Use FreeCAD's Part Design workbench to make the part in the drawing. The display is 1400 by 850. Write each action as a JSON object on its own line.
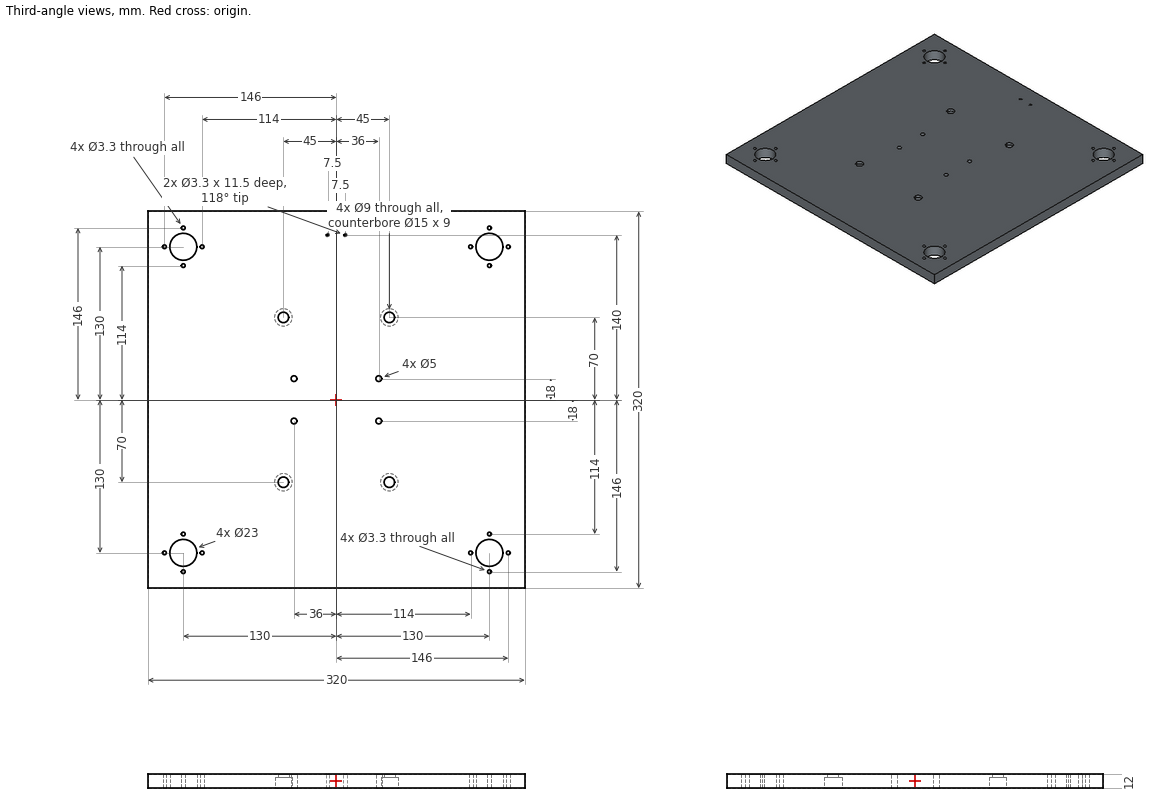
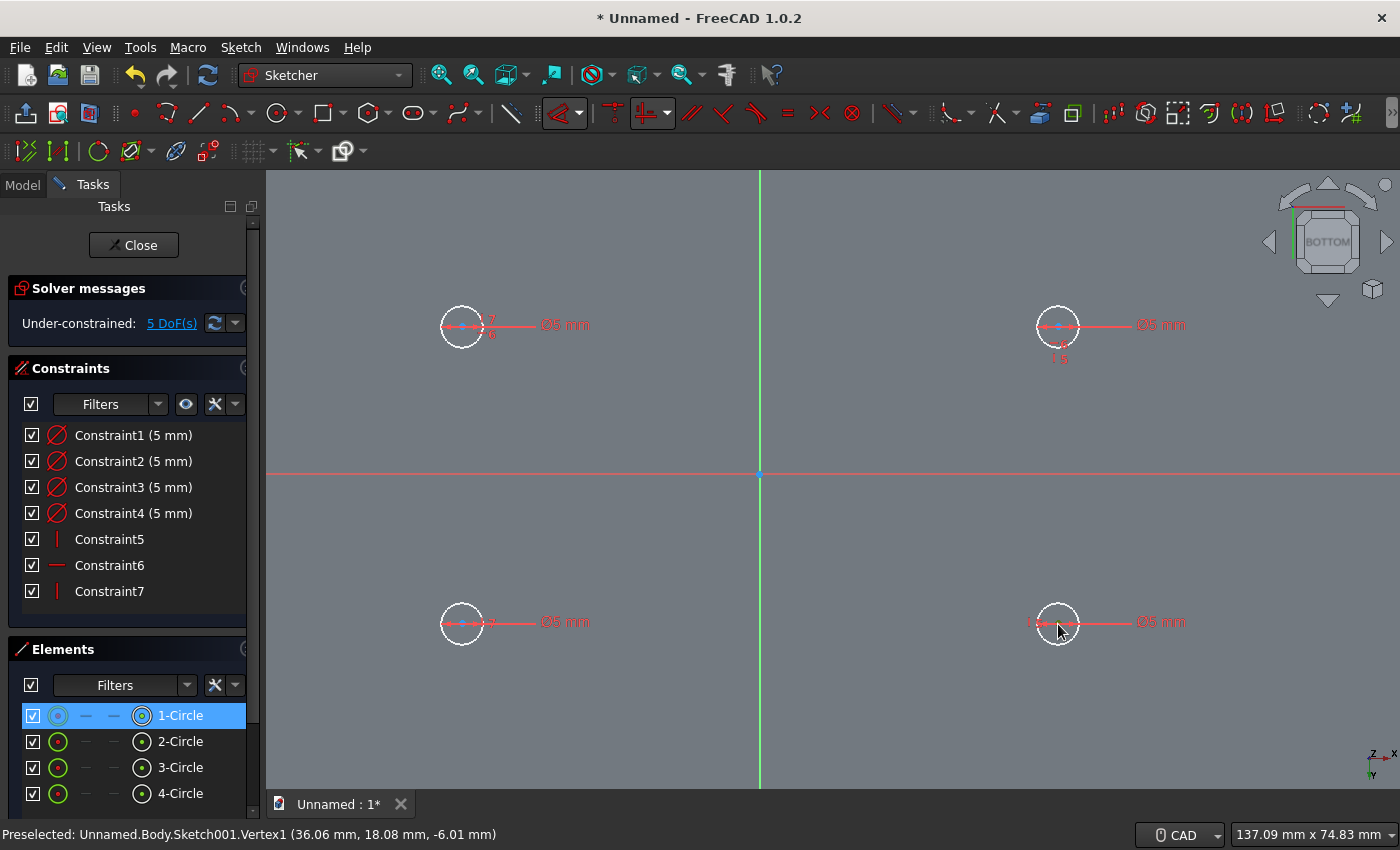
{"action": "left_click", "coordinate": [462, 624]}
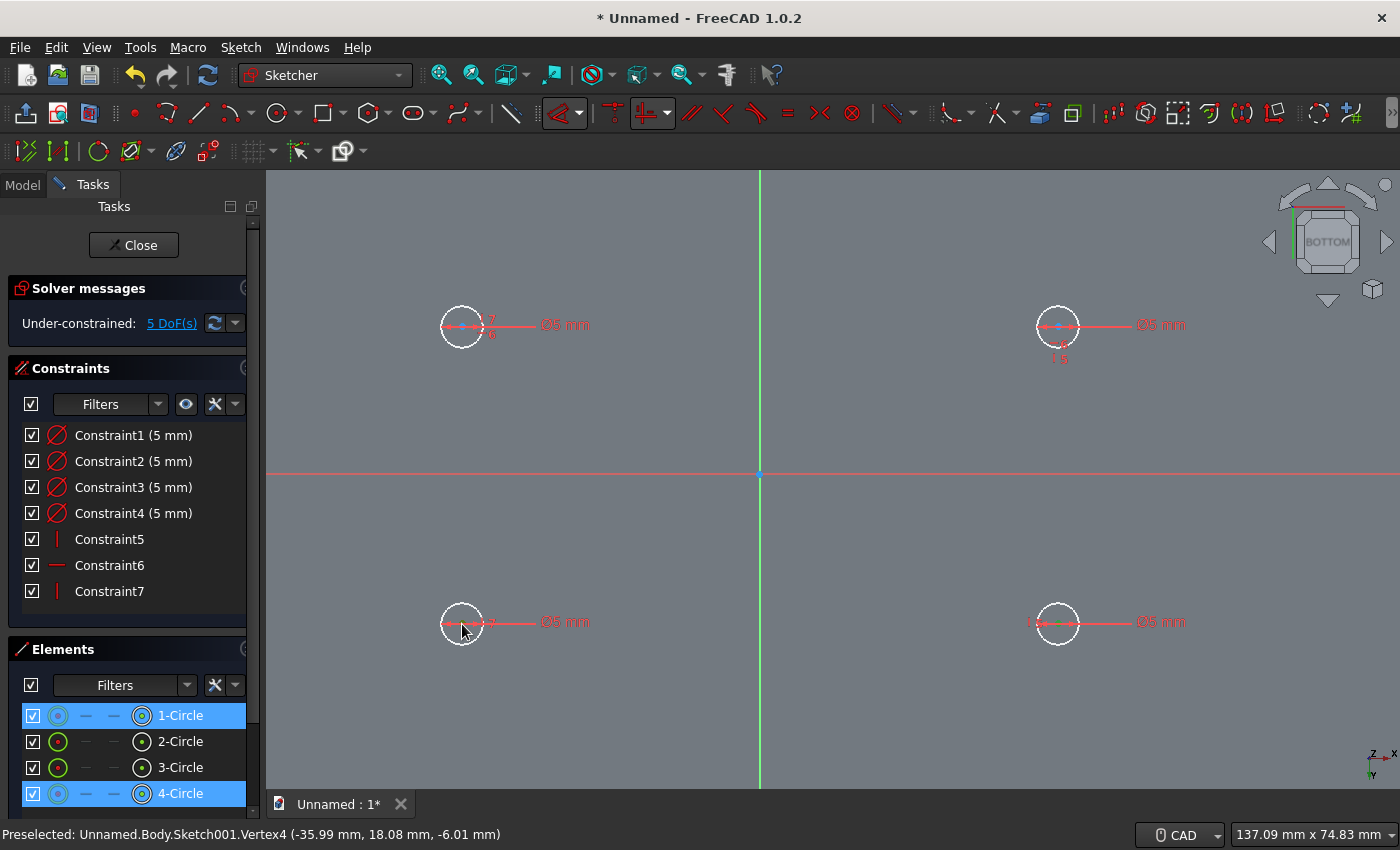
{"action": "key", "text": "h"}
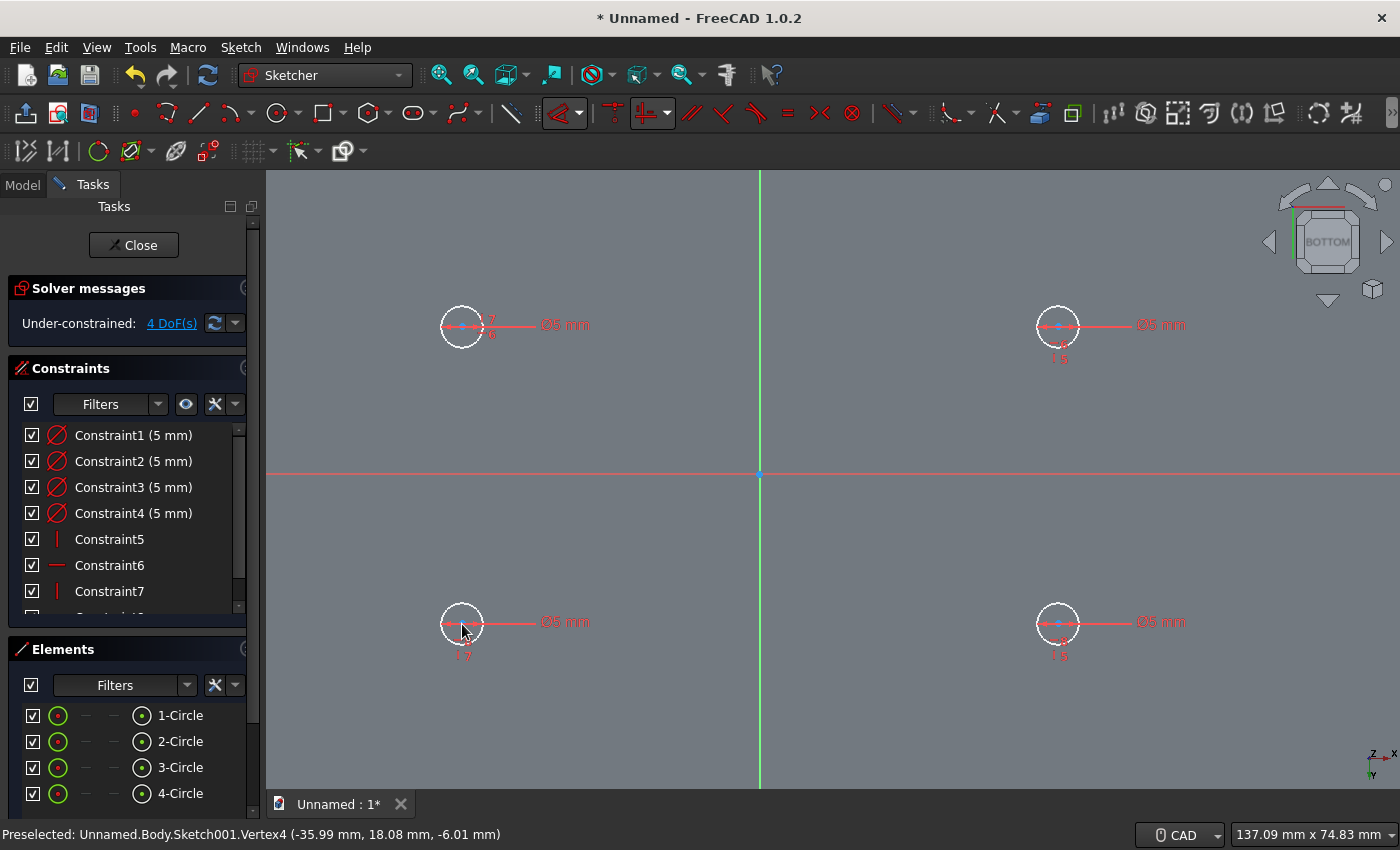
{"action": "left_click", "coordinate": [1058, 624]}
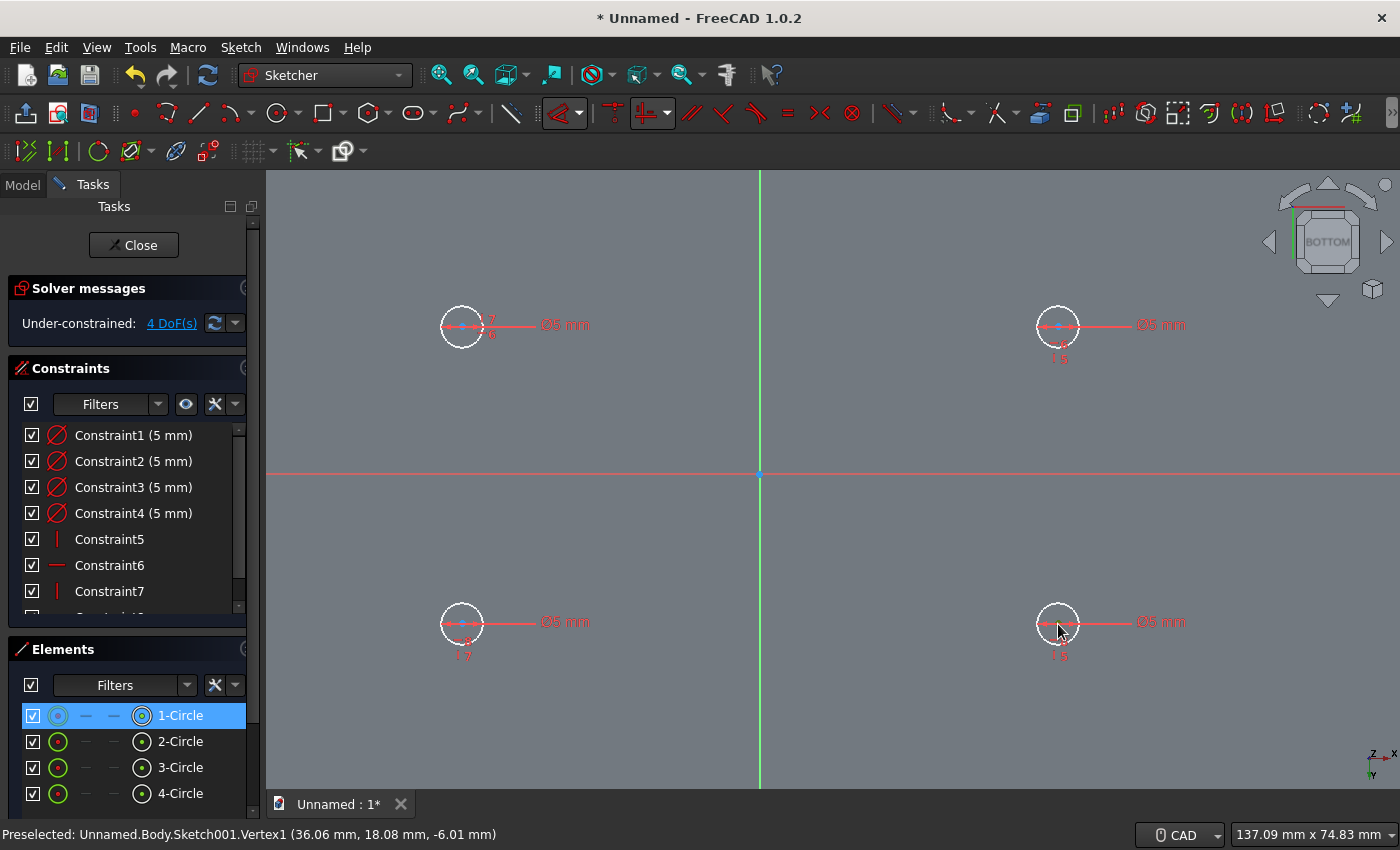
{"action": "left_click", "coordinate": [582, 114]}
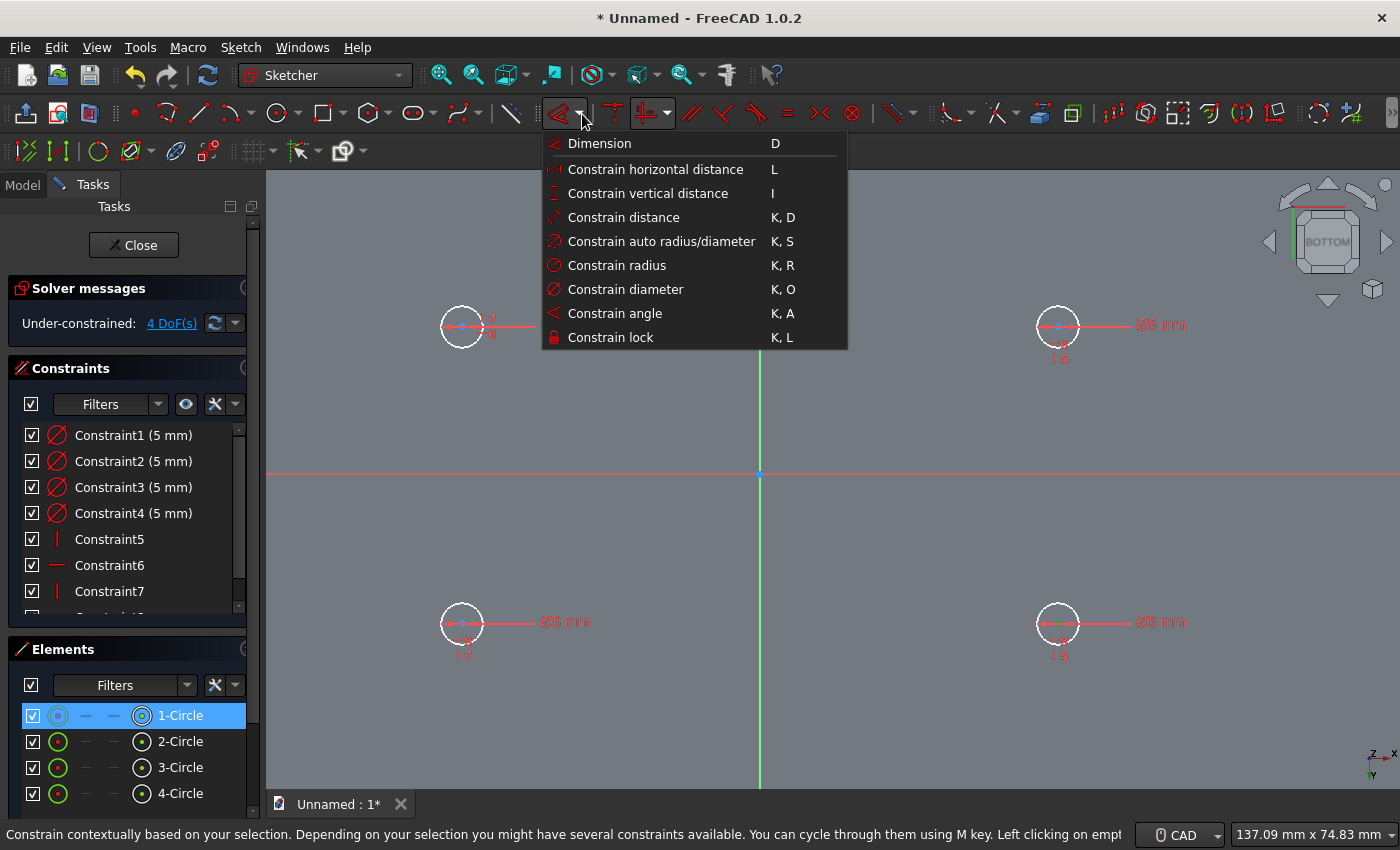
{"action": "left_click", "coordinate": [695, 169]}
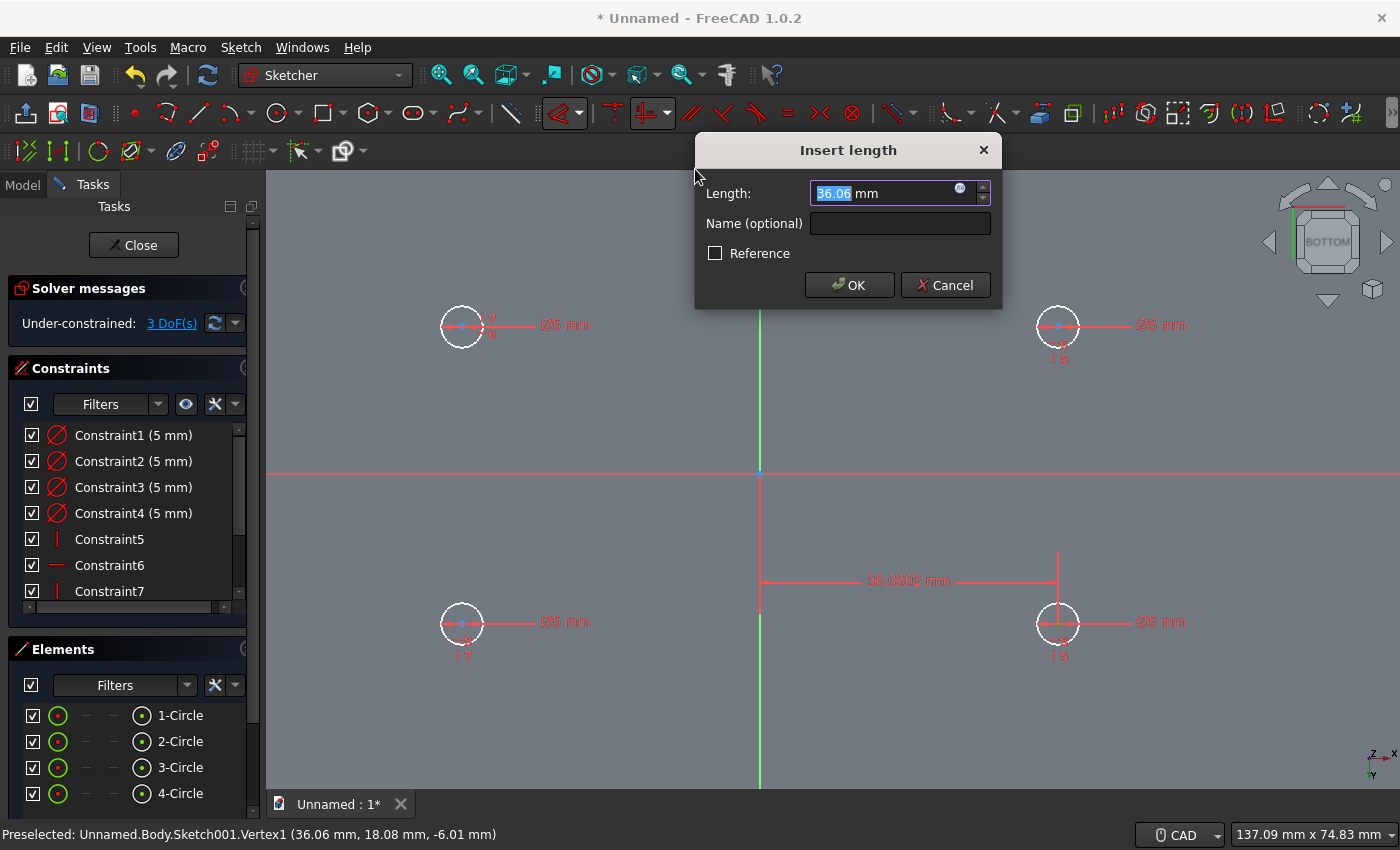
{"action": "type", "text": "36"}
{"action": "key", "text": "Return"}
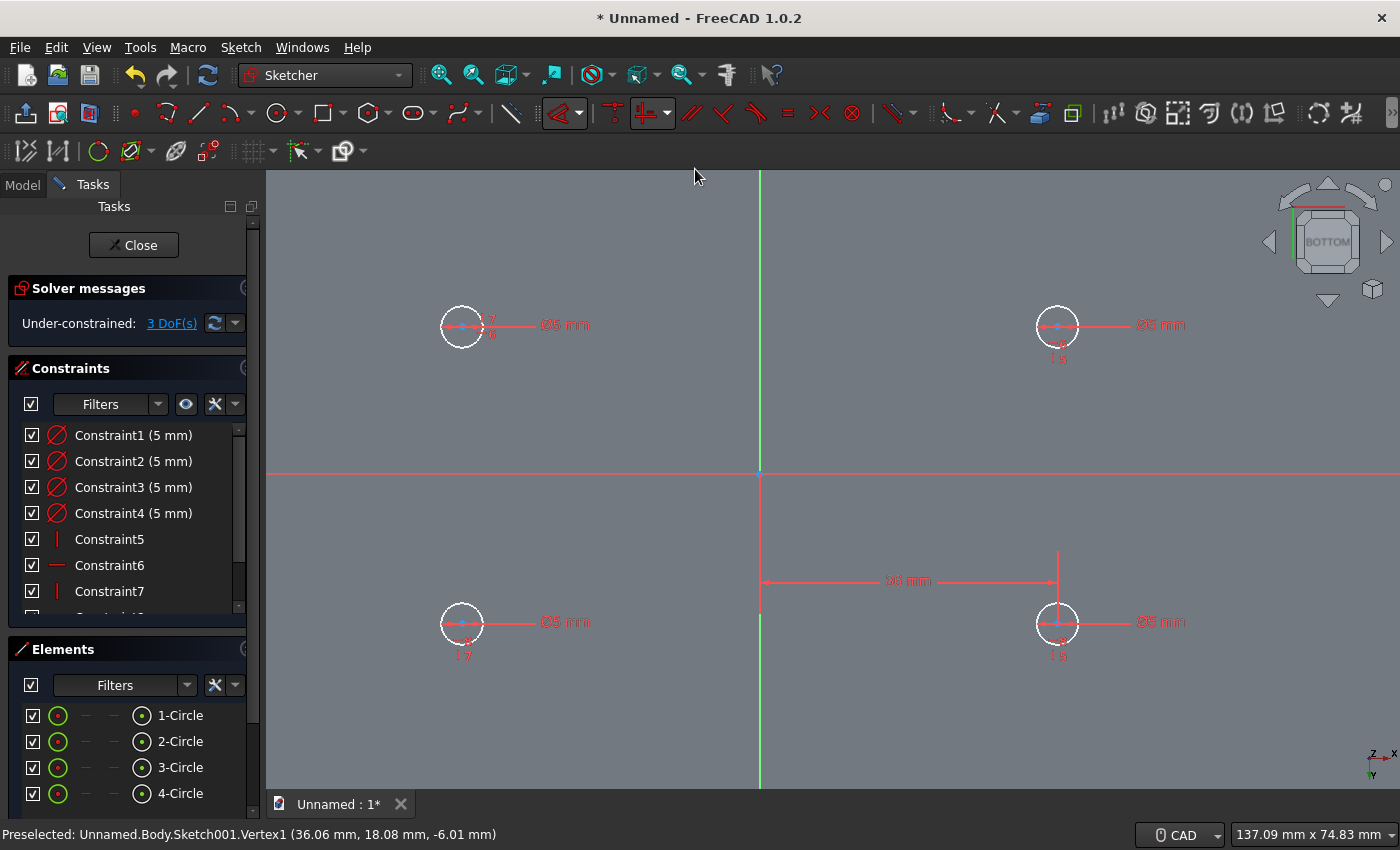
{"action": "left_click", "coordinate": [1058, 624]}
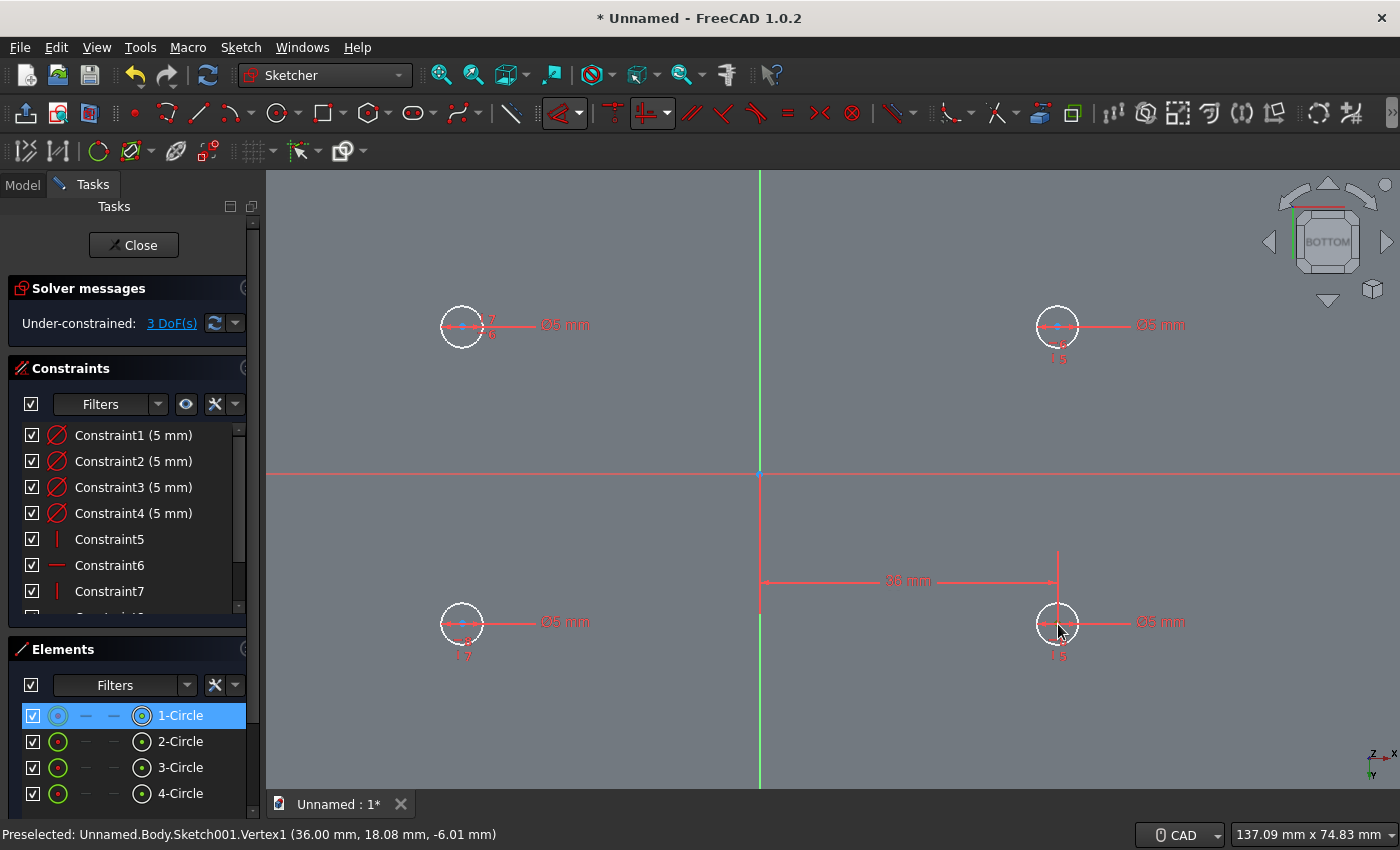
{"action": "left_click", "coordinate": [582, 114]}